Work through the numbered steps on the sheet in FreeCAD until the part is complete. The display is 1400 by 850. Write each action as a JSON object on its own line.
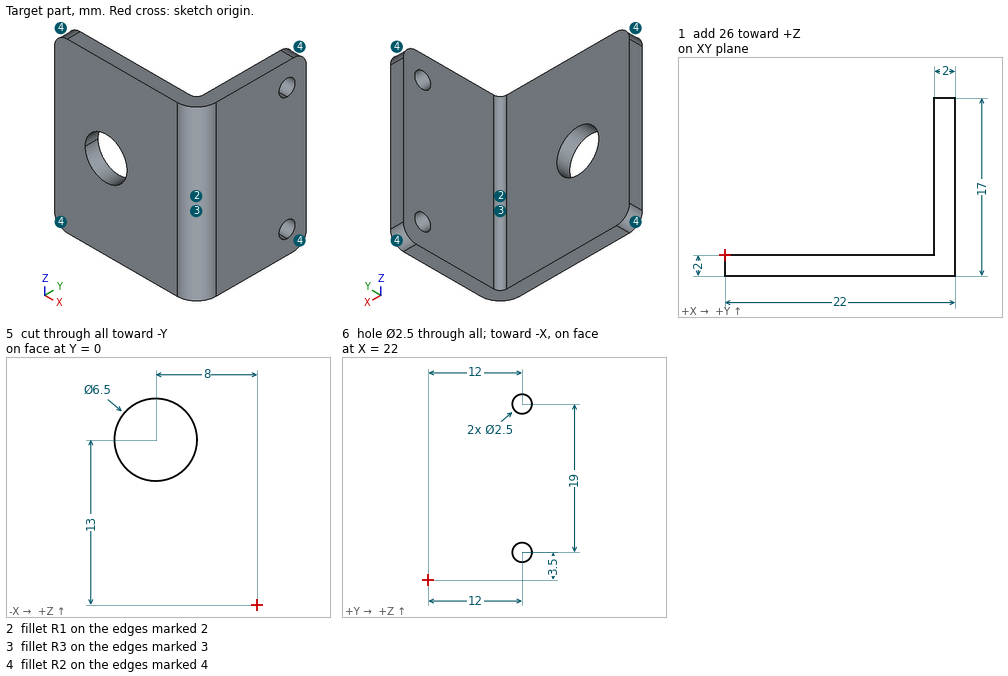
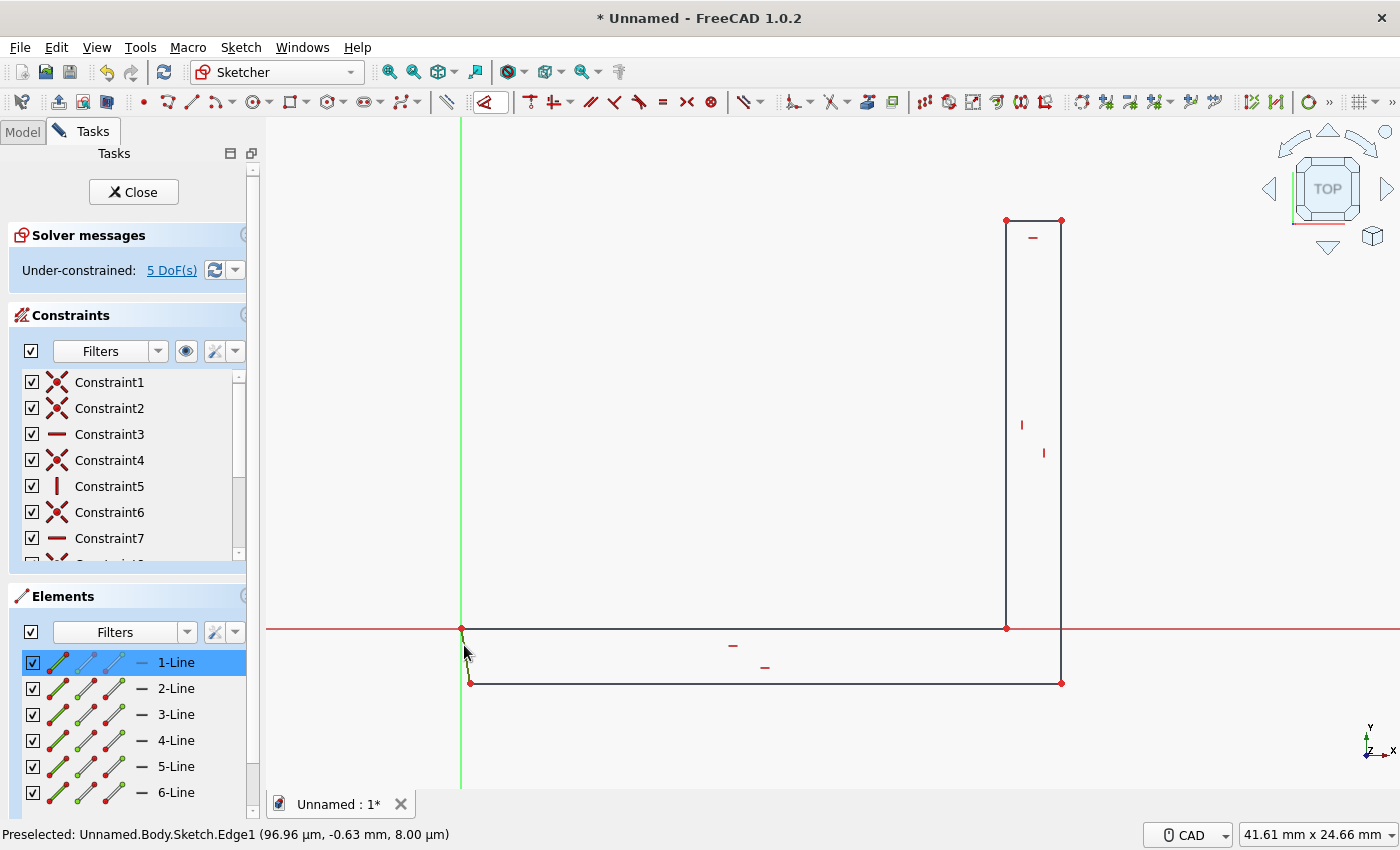
{"action": "key", "text": "v"}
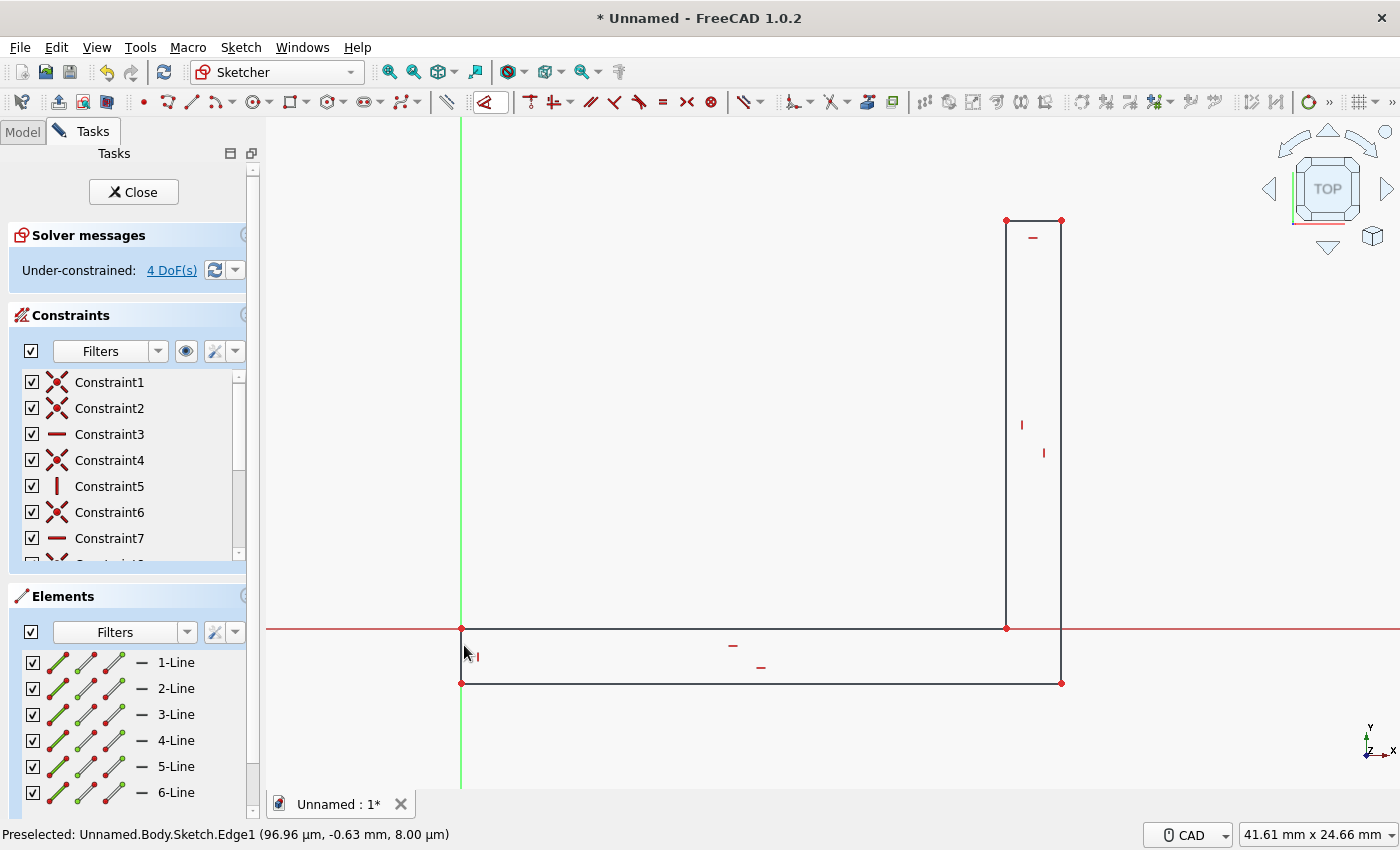
{"action": "key", "text": "d"}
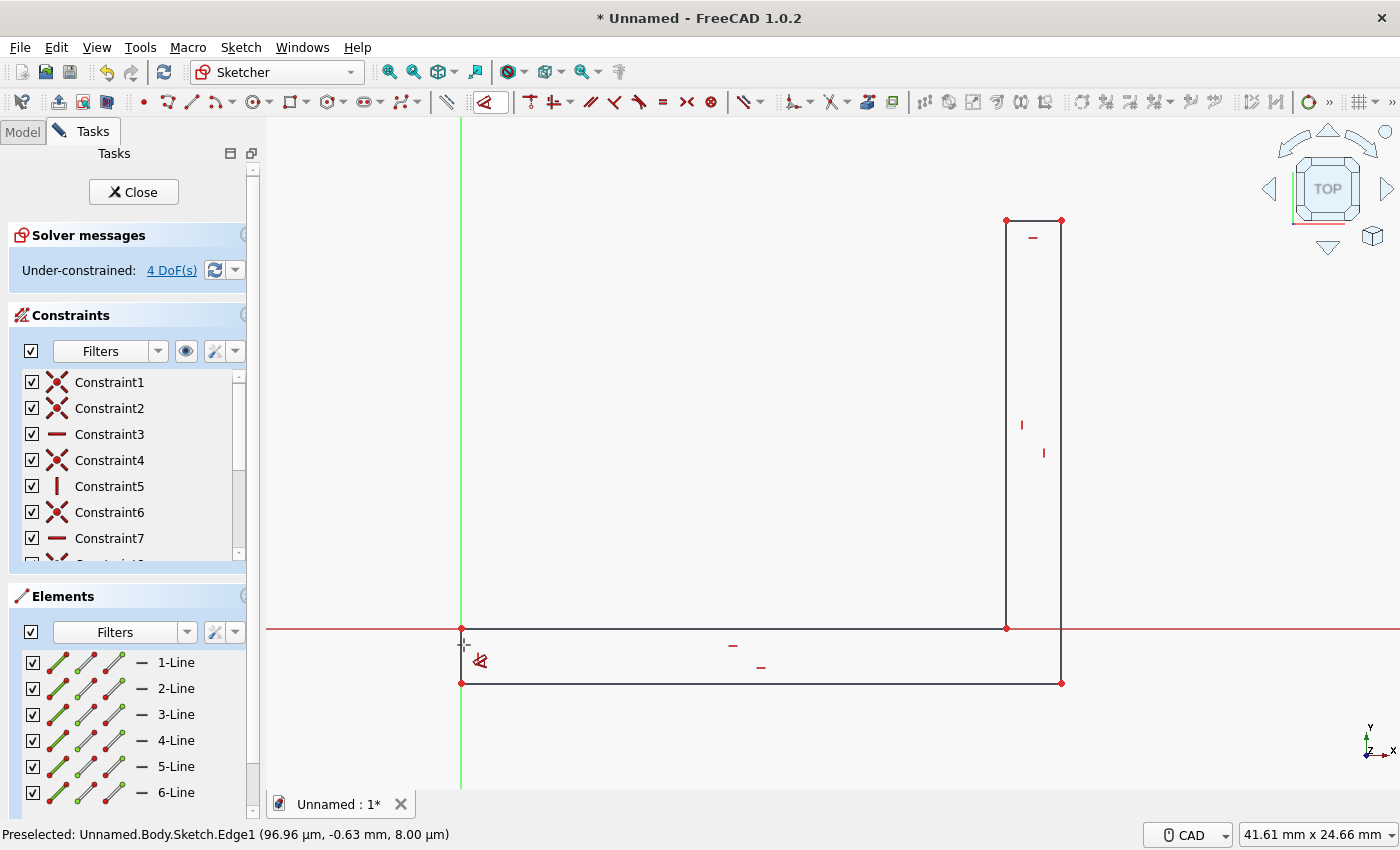
{"action": "left_click", "coordinate": [461, 645]}
{"action": "left_click", "coordinate": [427, 656]}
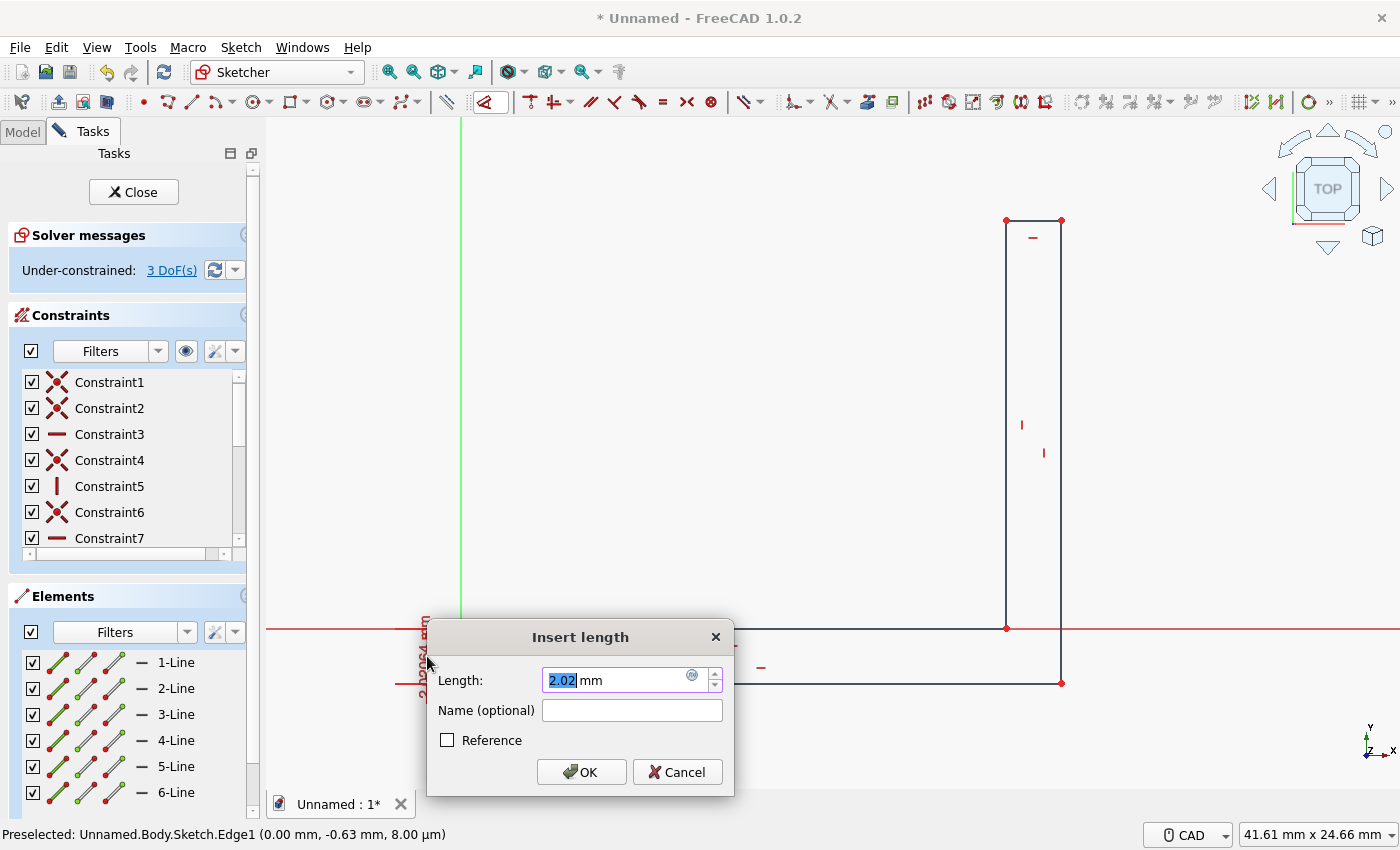
{"action": "type", "text": "2"}
{"action": "key", "text": "Return"}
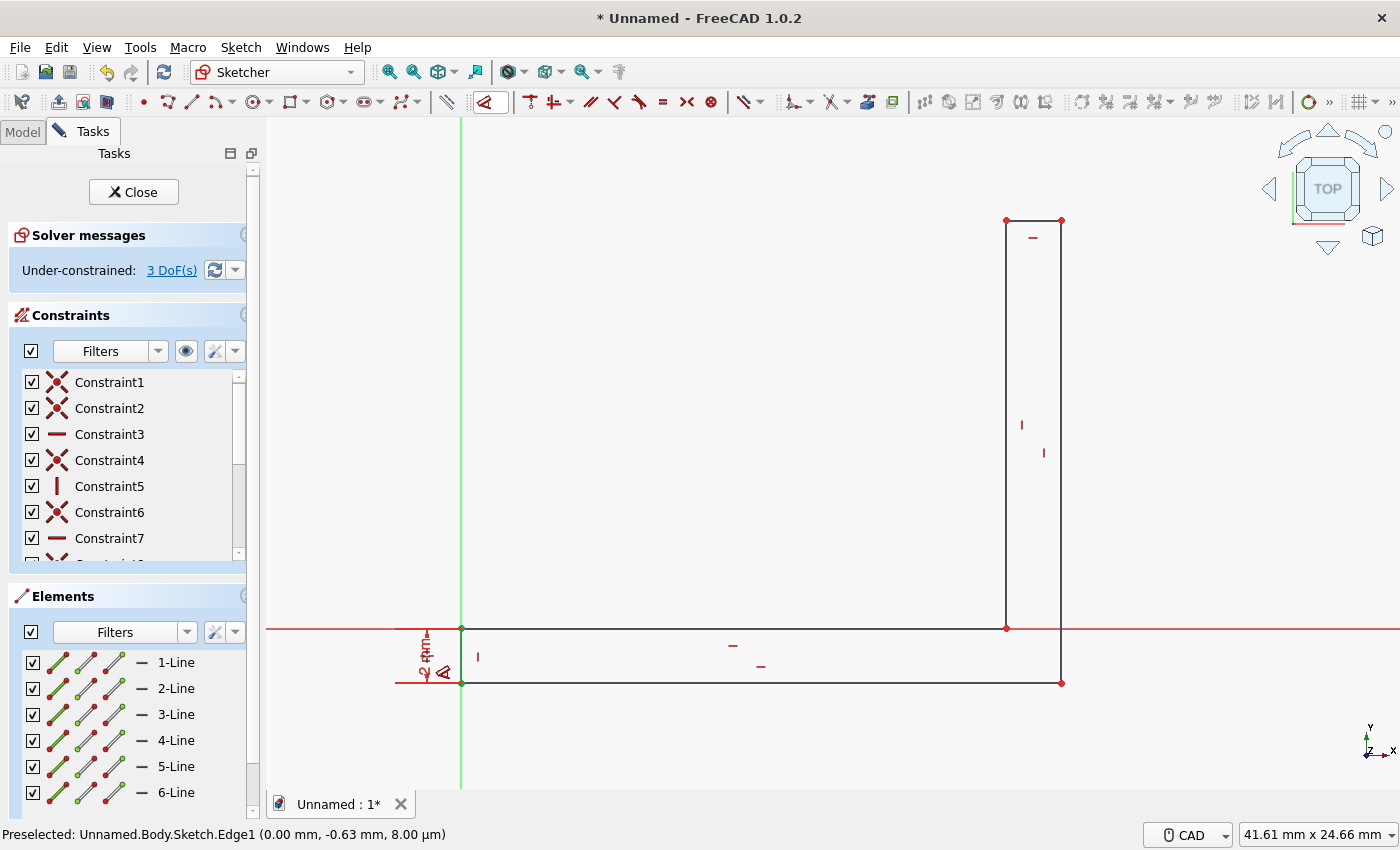
{"action": "left_click", "coordinate": [1044, 221]}
{"action": "left_click", "coordinate": [1033, 187]}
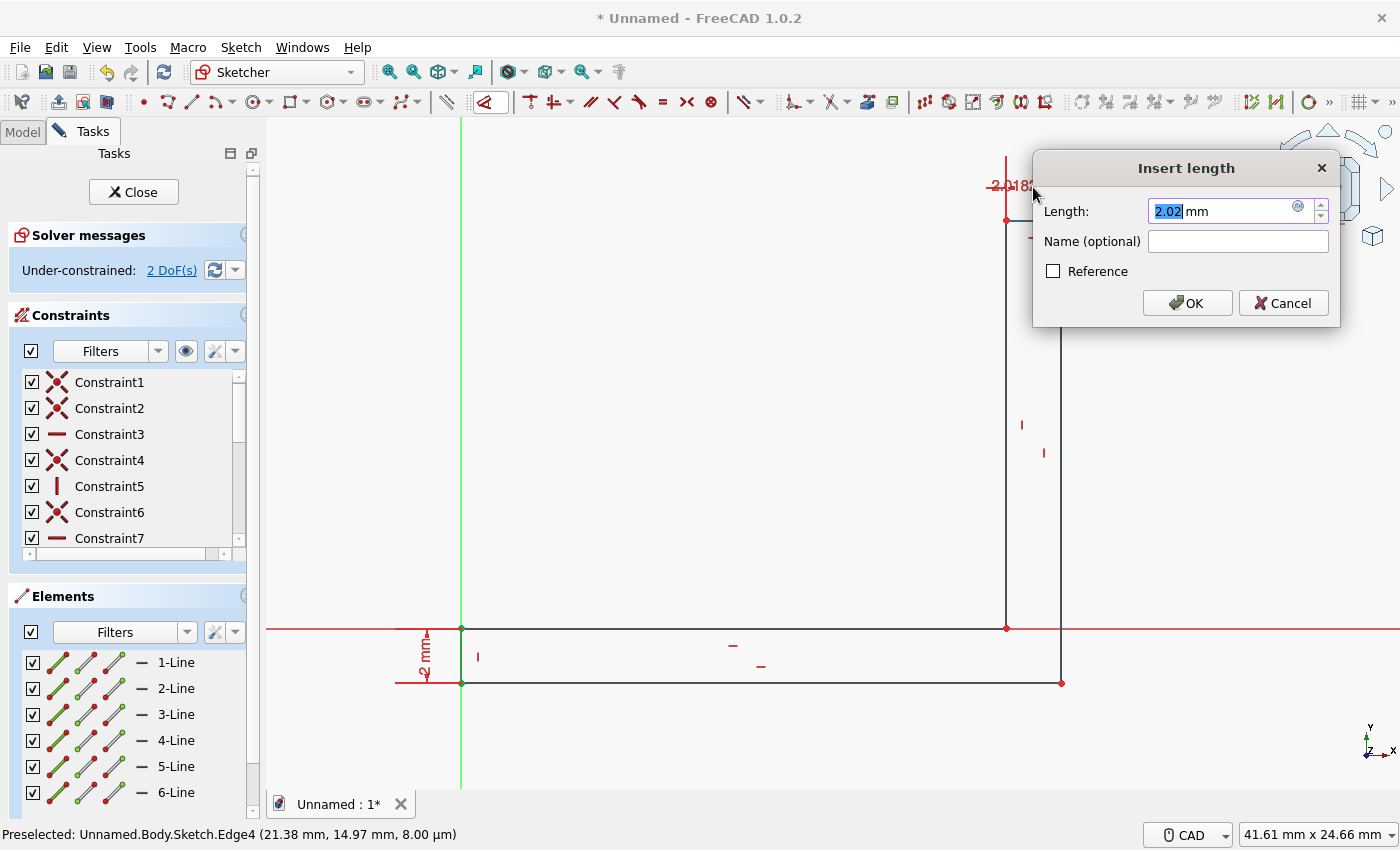
{"action": "type", "text": "2"}
{"action": "key", "text": "Return"}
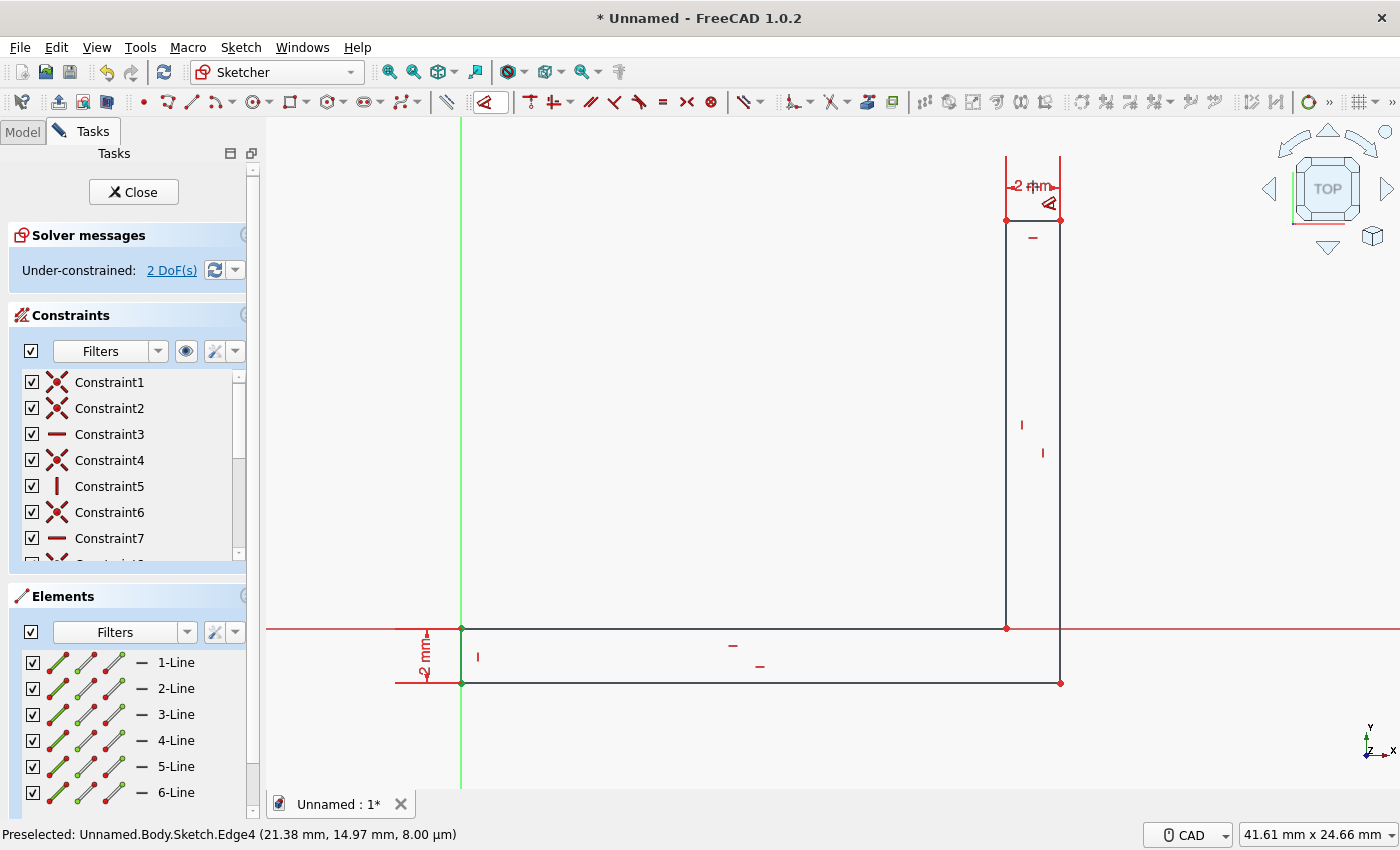
{"action": "left_click", "coordinate": [641, 683]}
{"action": "left_click", "coordinate": [761, 717]}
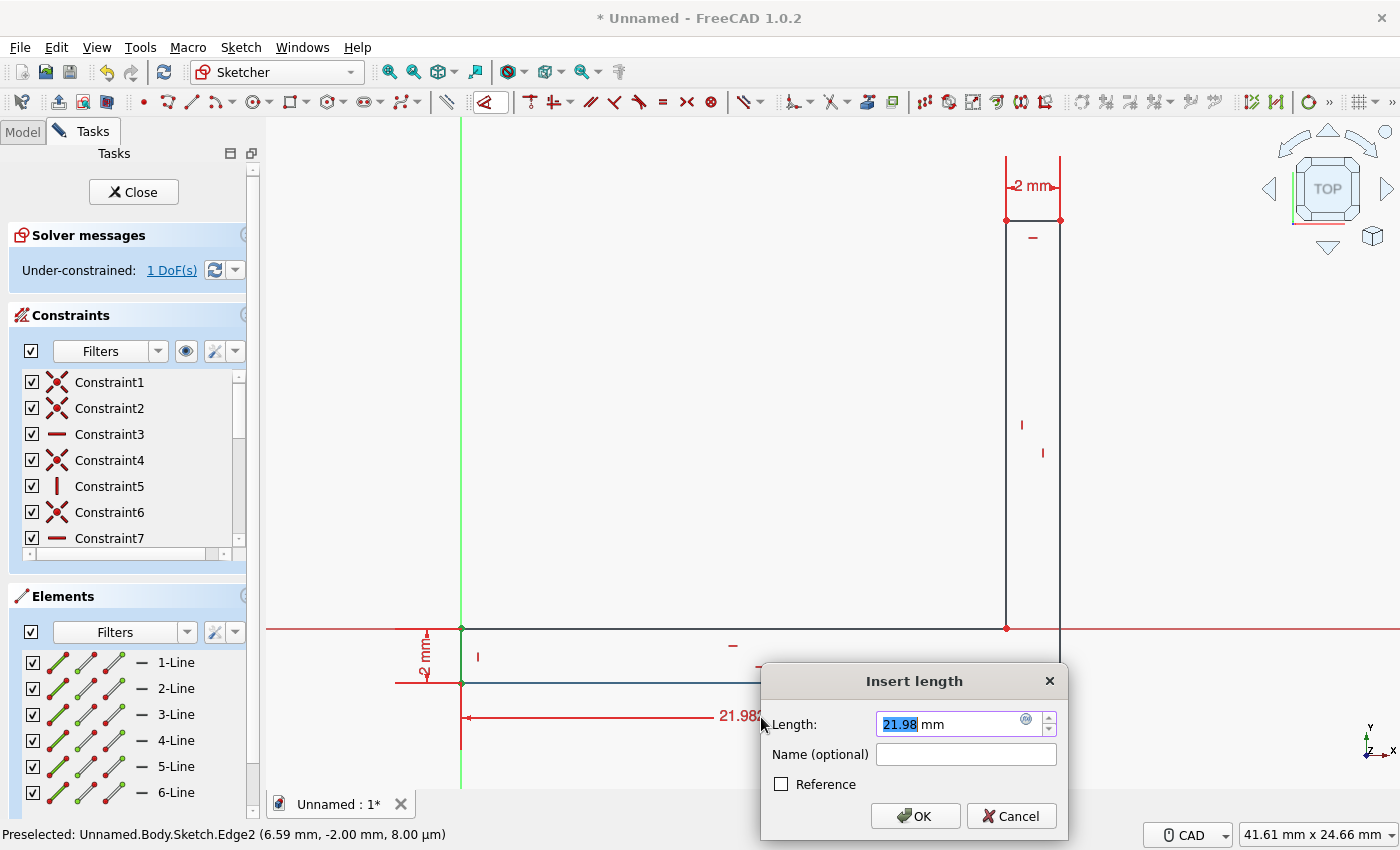
{"action": "type", "text": "22"}
{"action": "key", "text": "Return"}